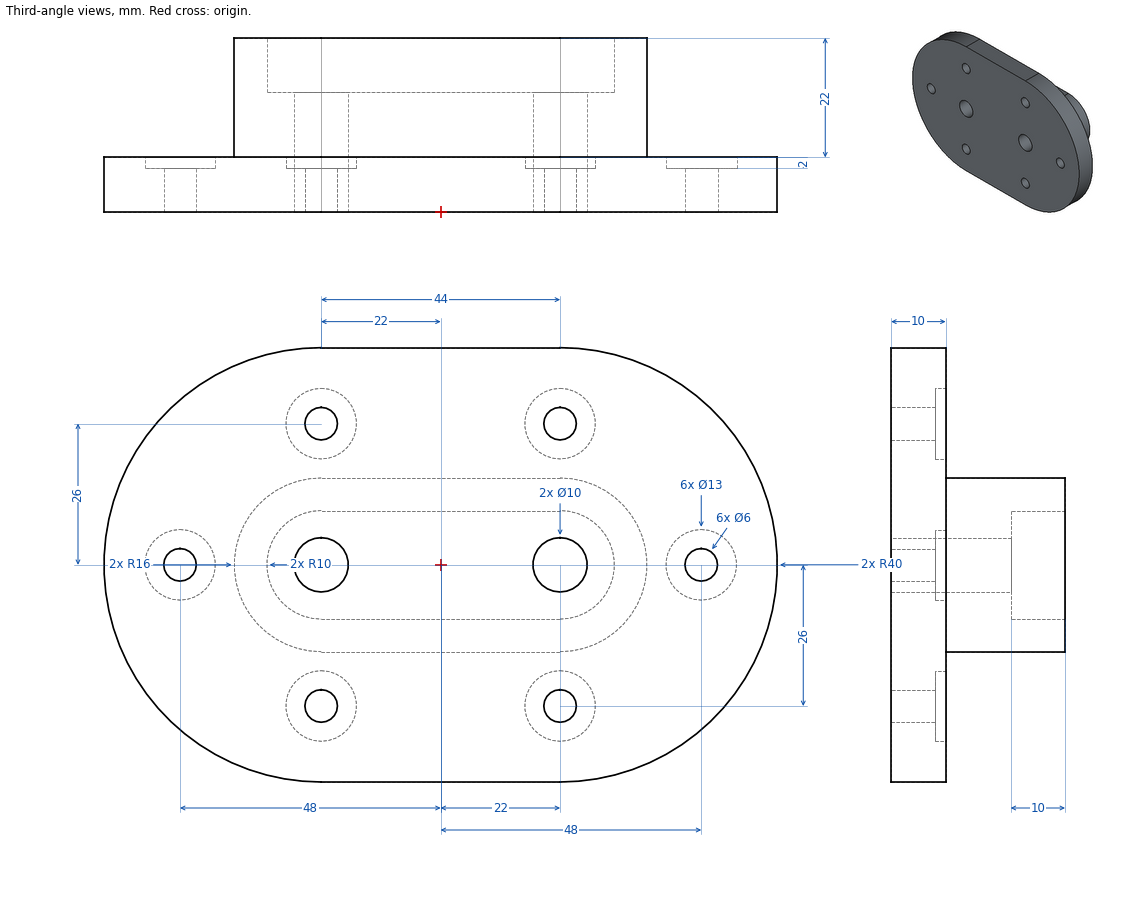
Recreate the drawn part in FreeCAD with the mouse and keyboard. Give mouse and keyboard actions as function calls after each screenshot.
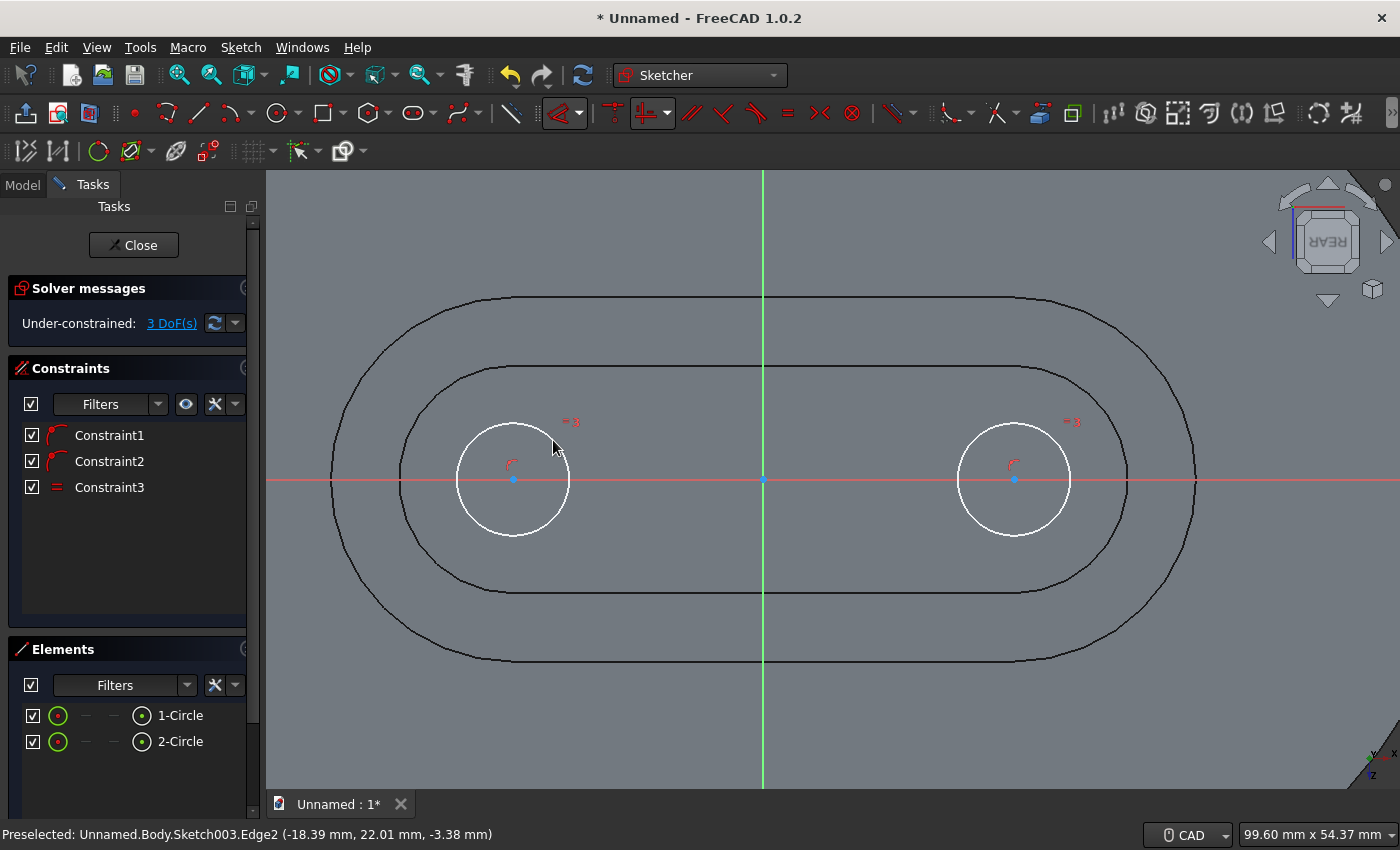
click(1054, 440)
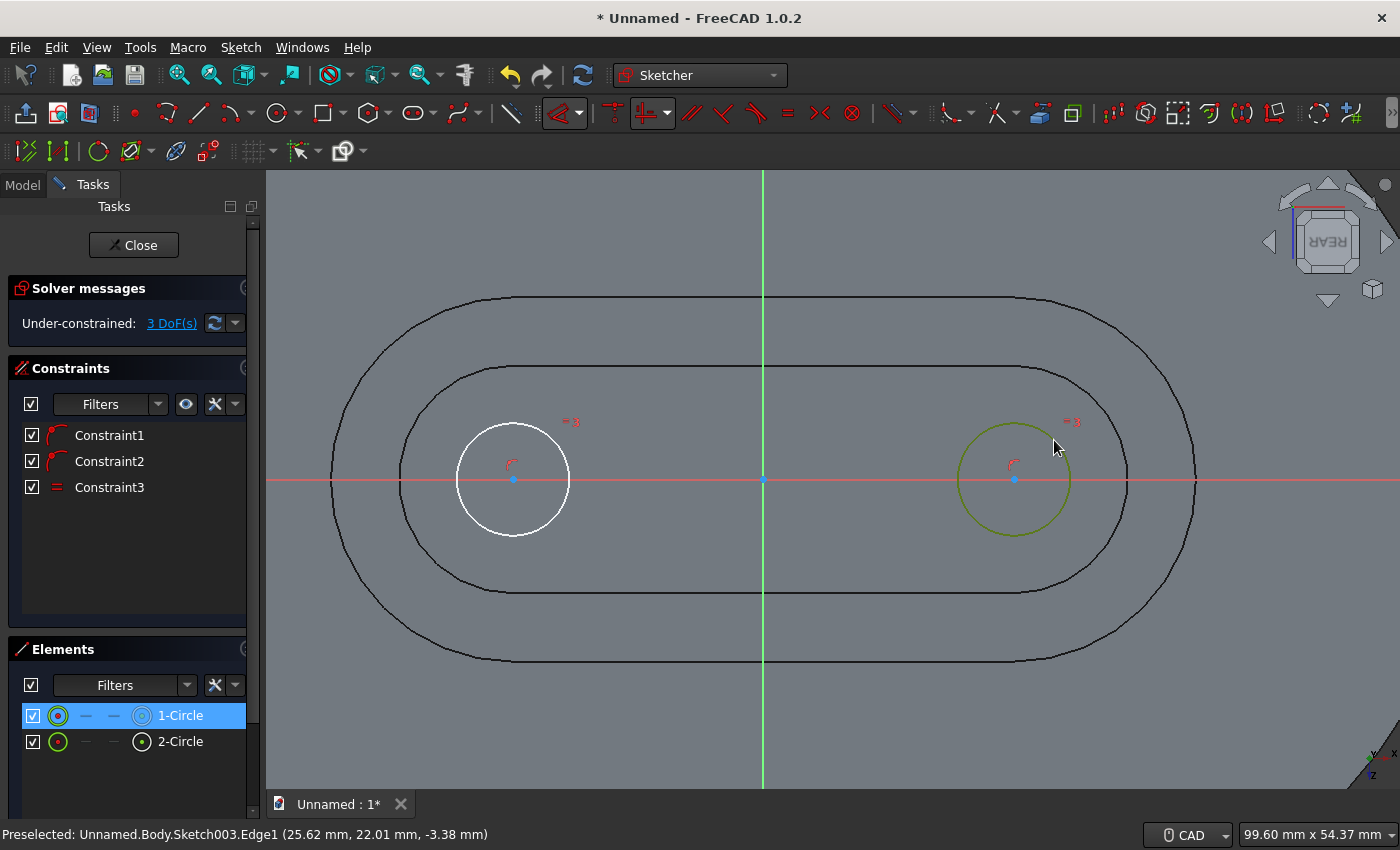
key(k)
key(o)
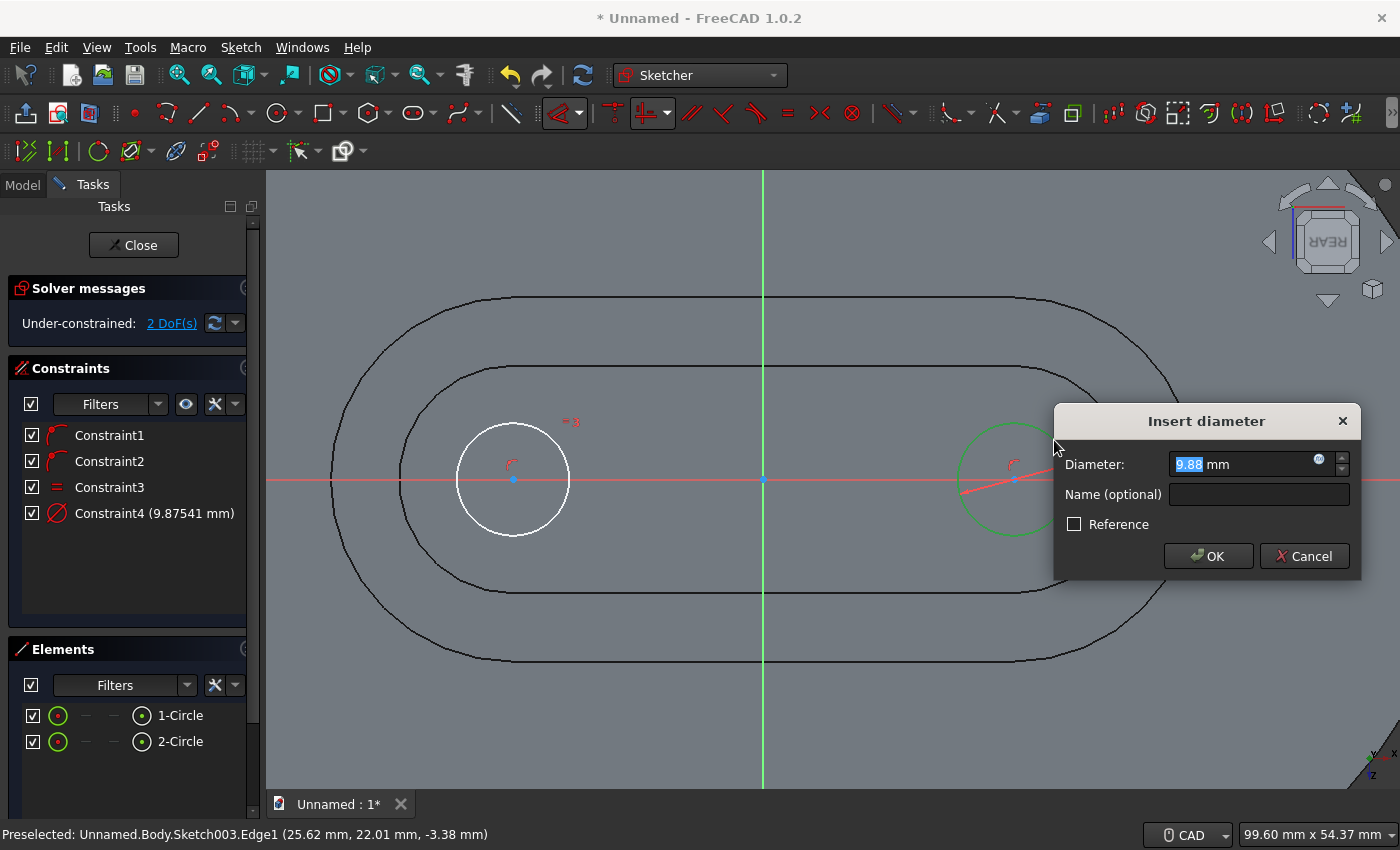
text(10)
key(Return)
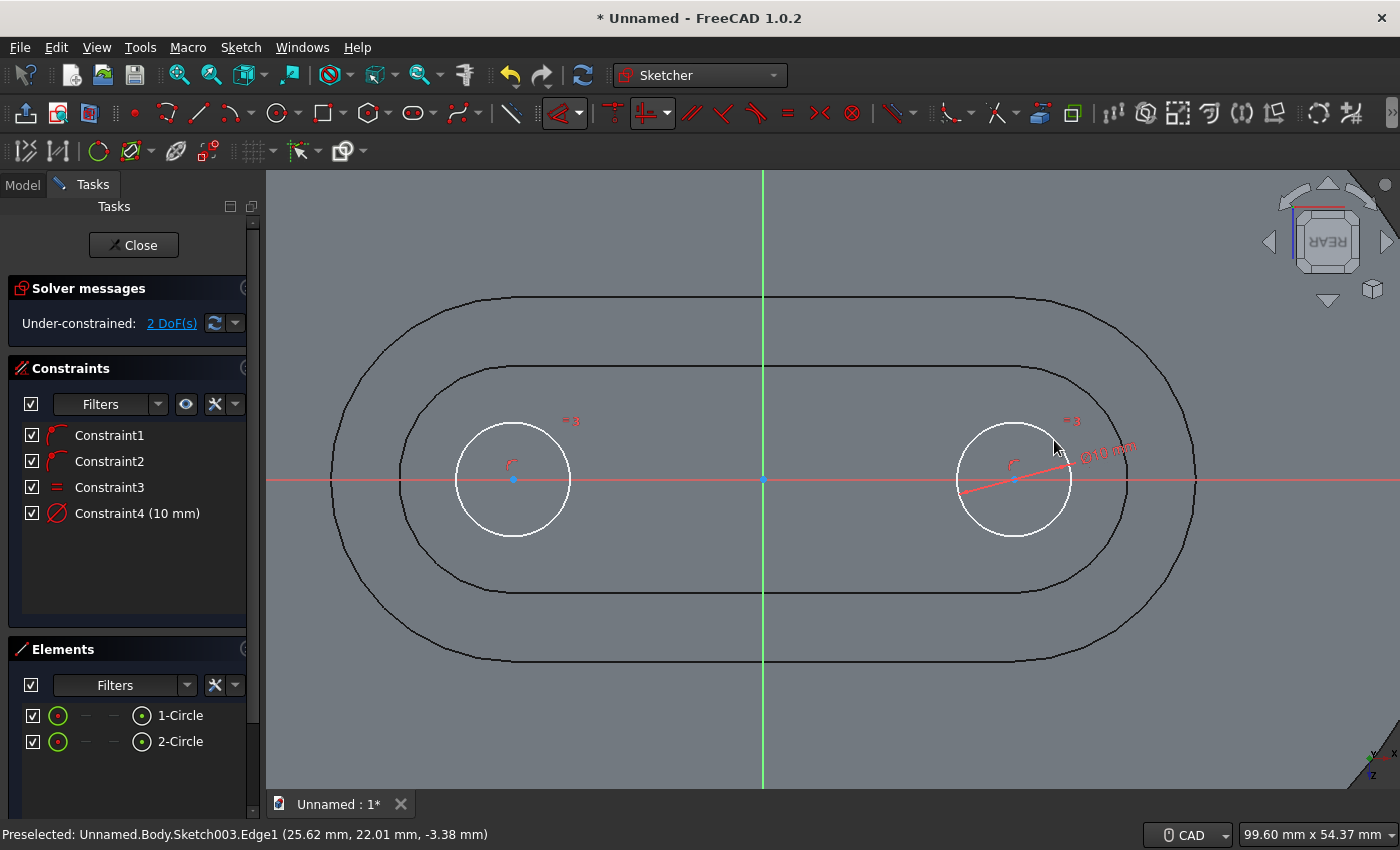
click(1014, 479)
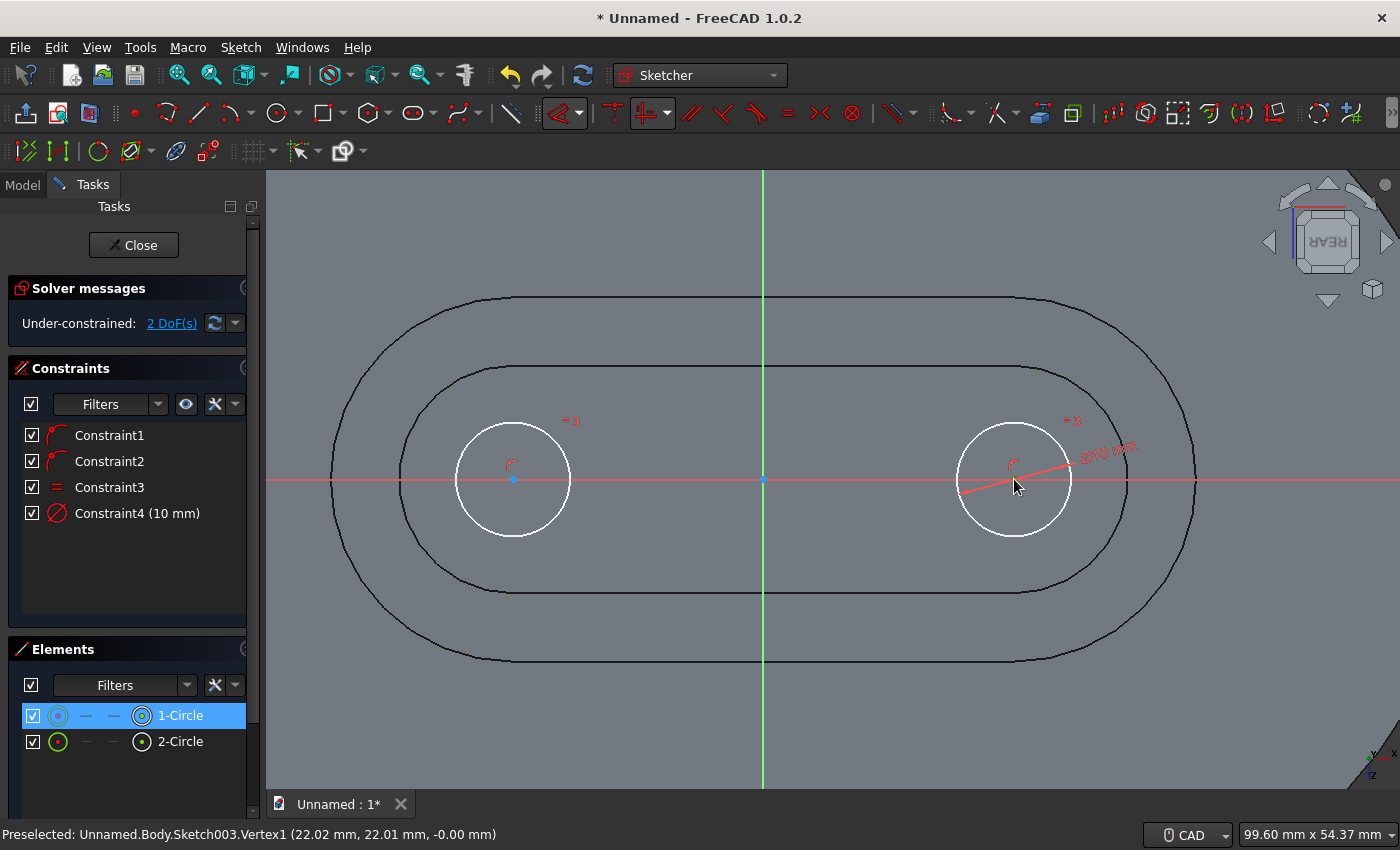
key(l)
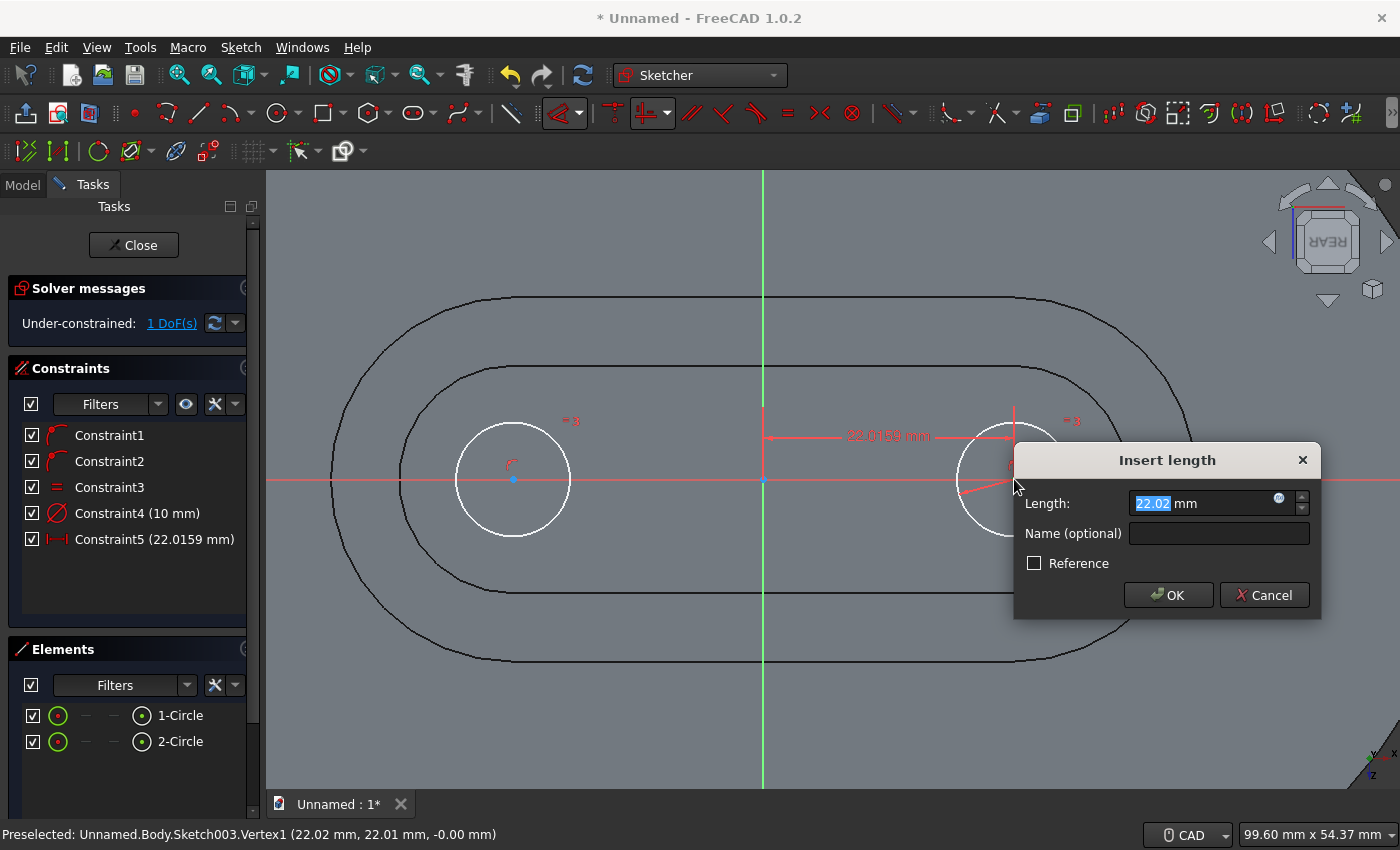
text(22)
key(Return)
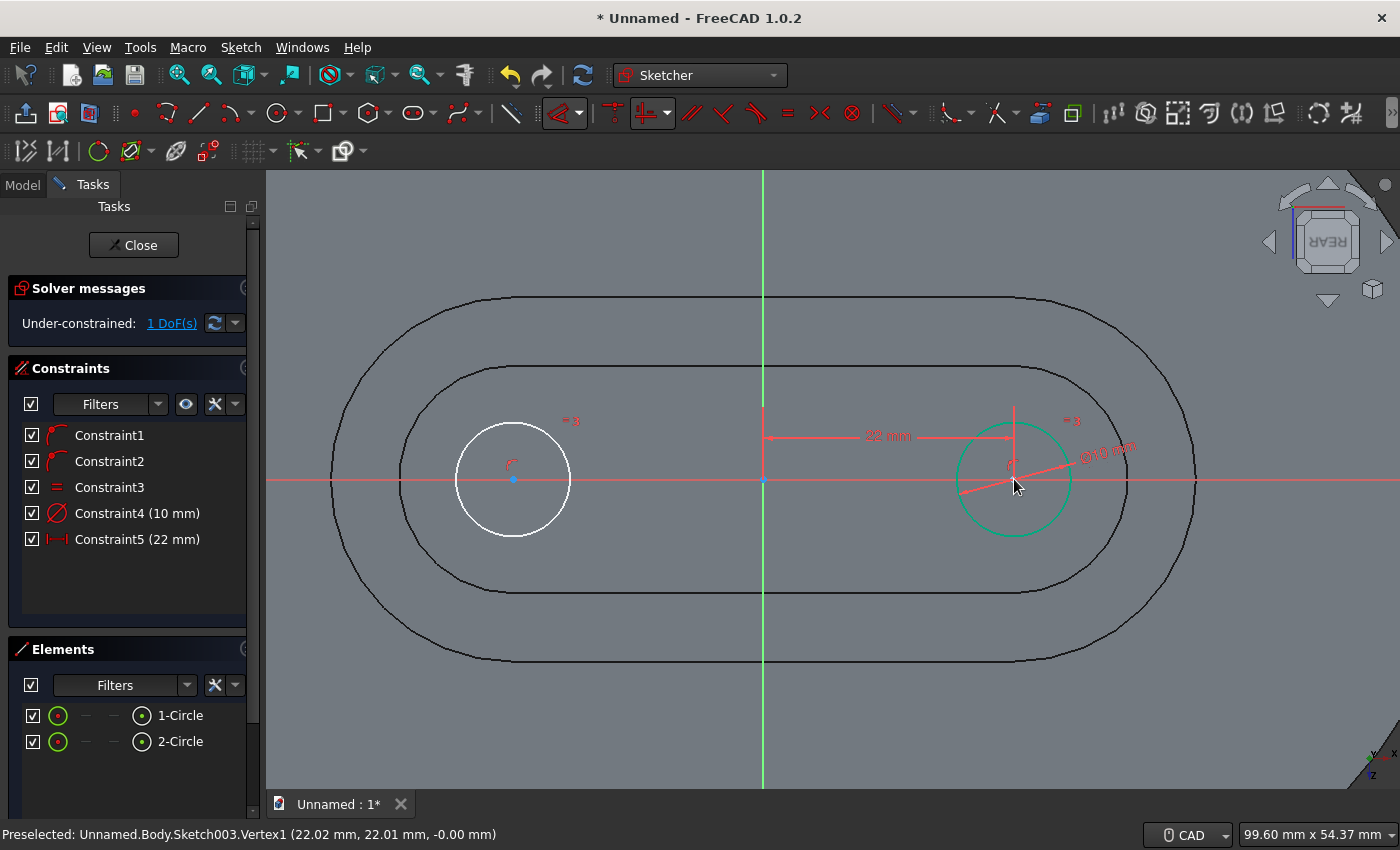
click(513, 479)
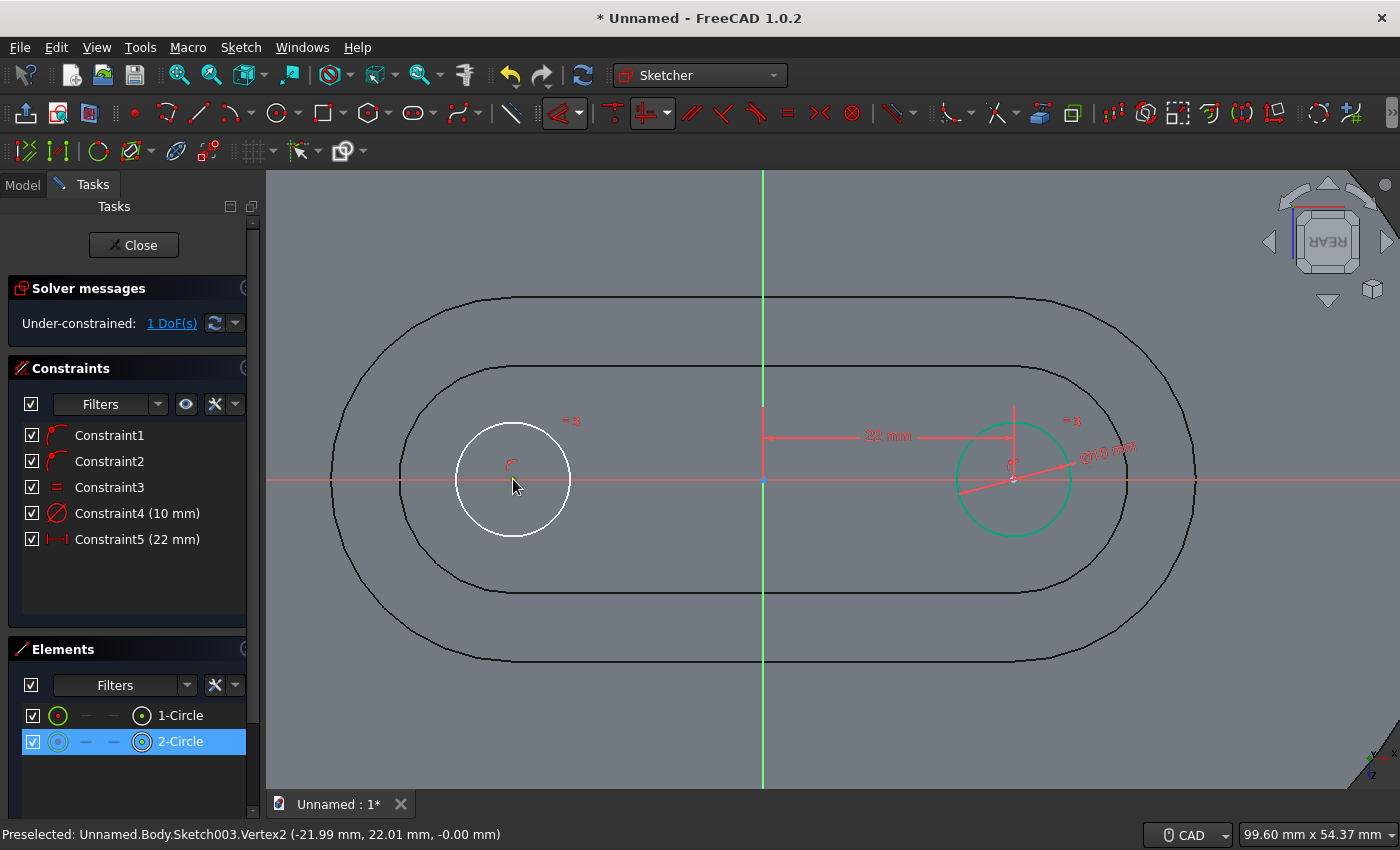
click(582, 114)